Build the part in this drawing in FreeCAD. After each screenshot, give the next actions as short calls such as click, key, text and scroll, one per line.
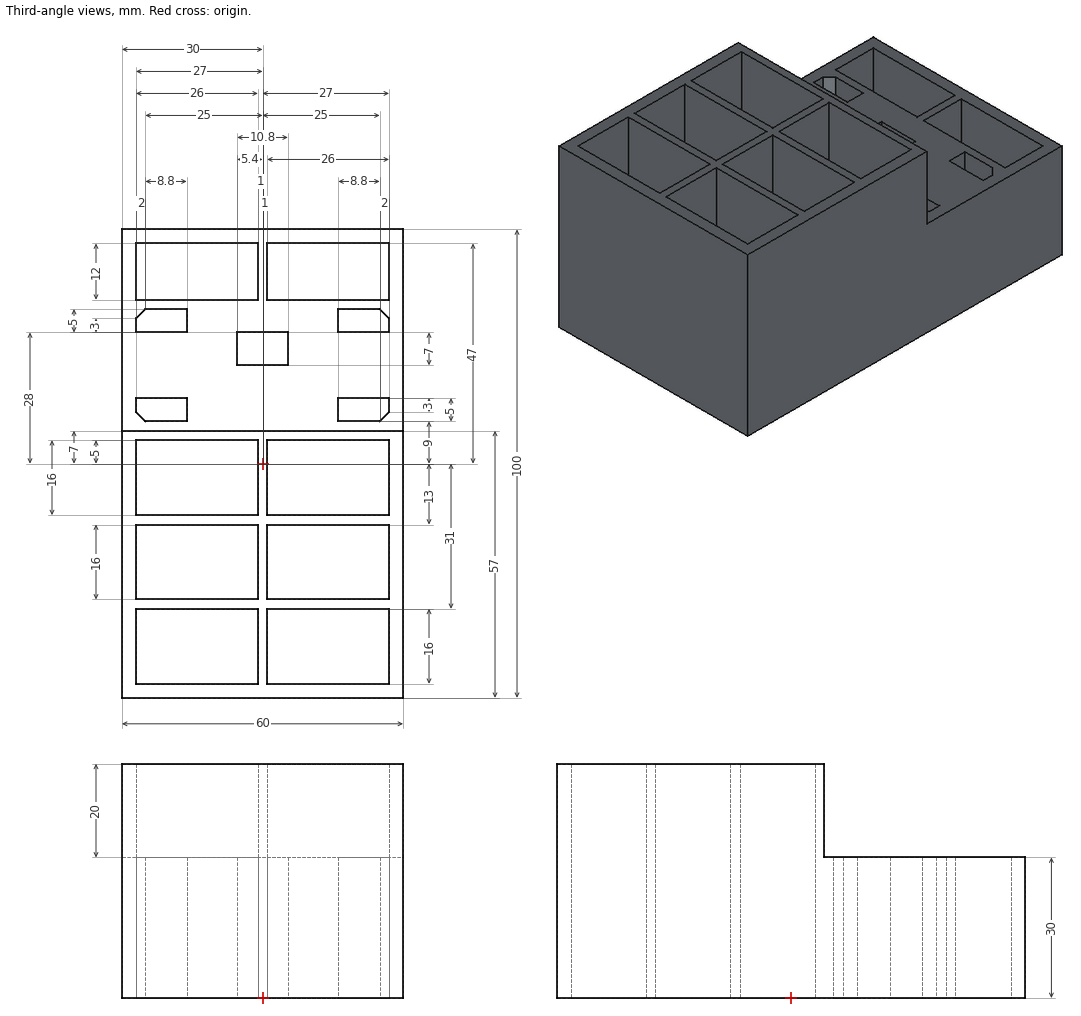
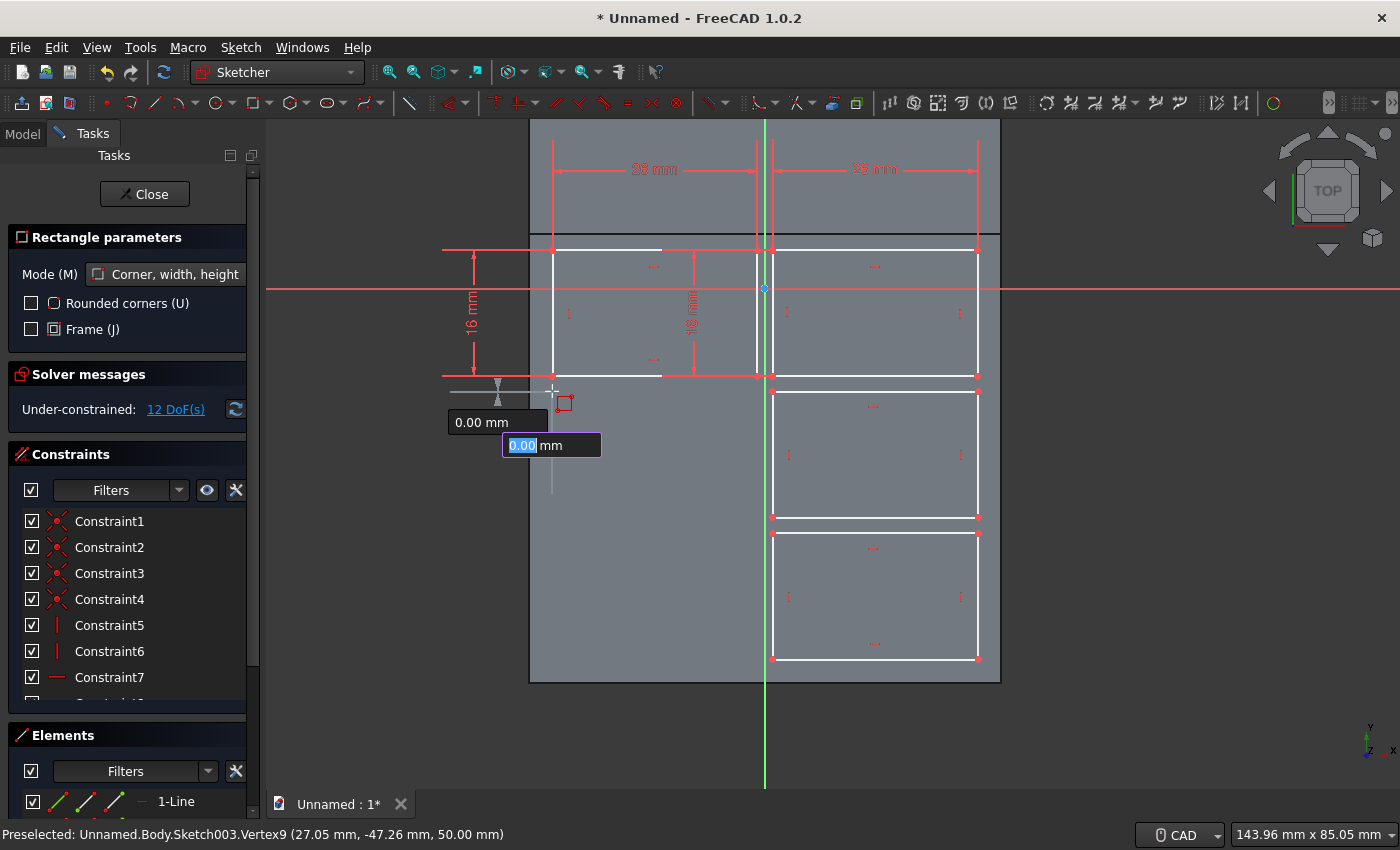
scroll(757, 517, up, 4)
move(756, 517)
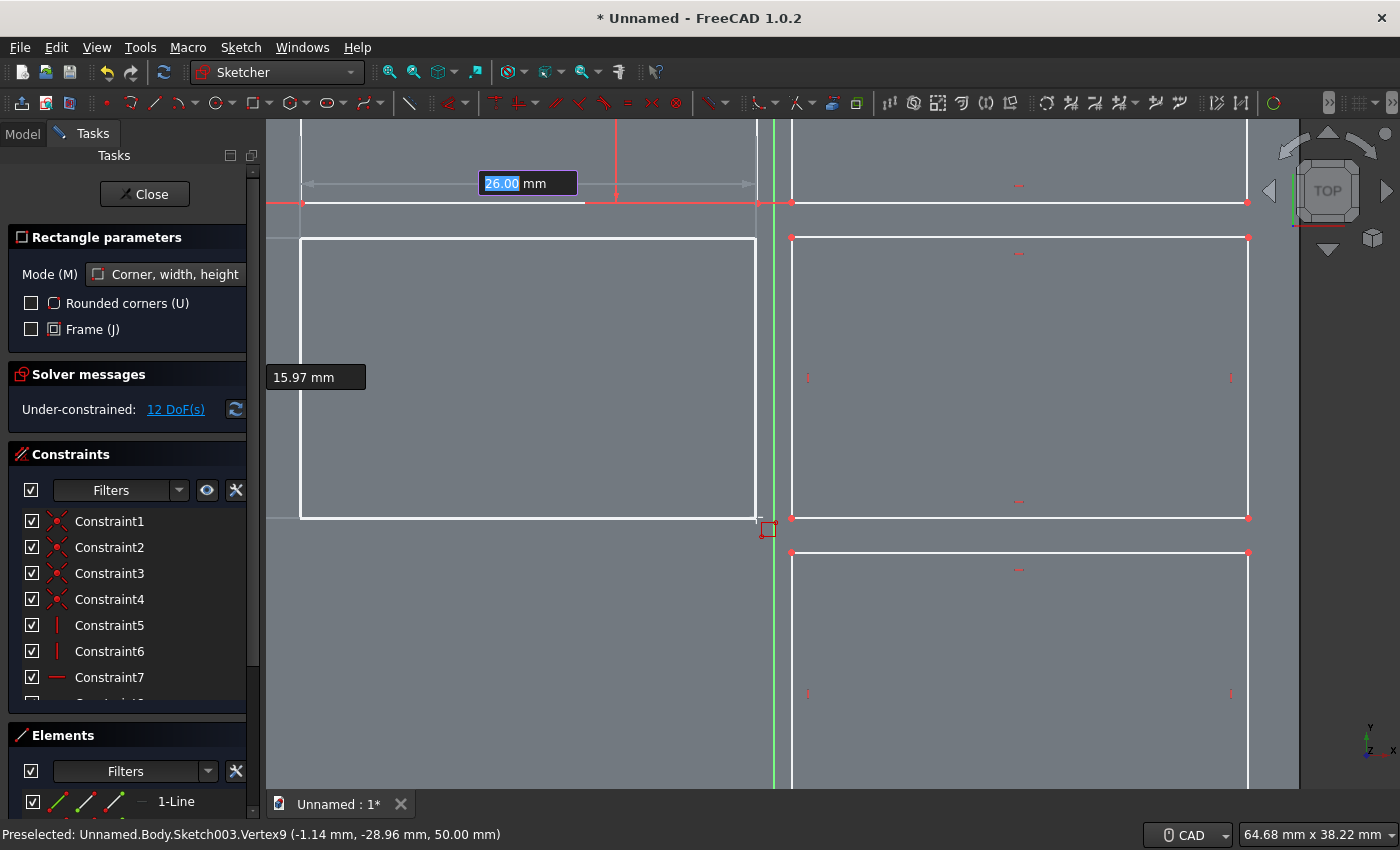
text(26)
key(Tab)
text(16)
key(Return)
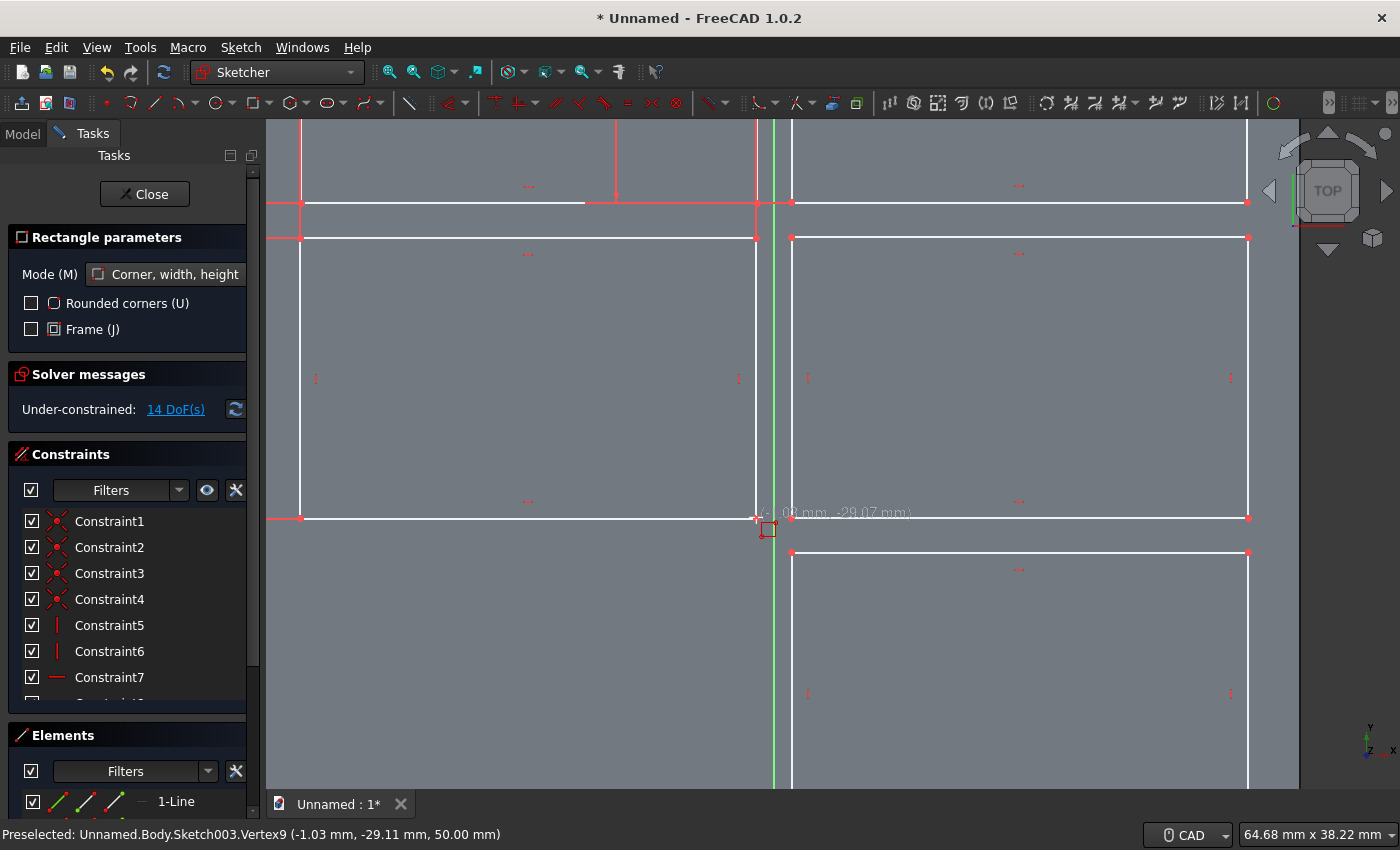
click(301, 552)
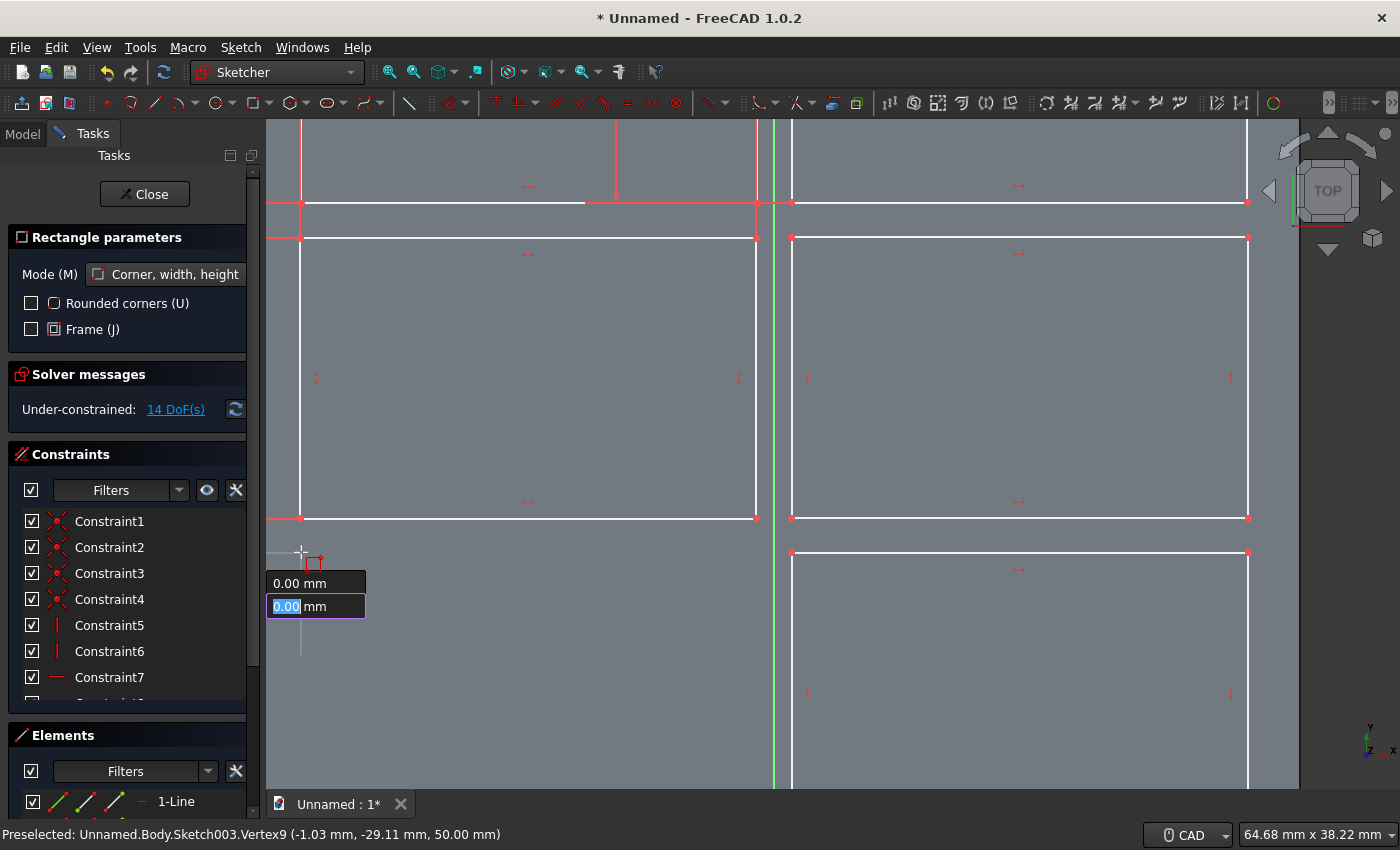
scroll(757, 517, down, 4)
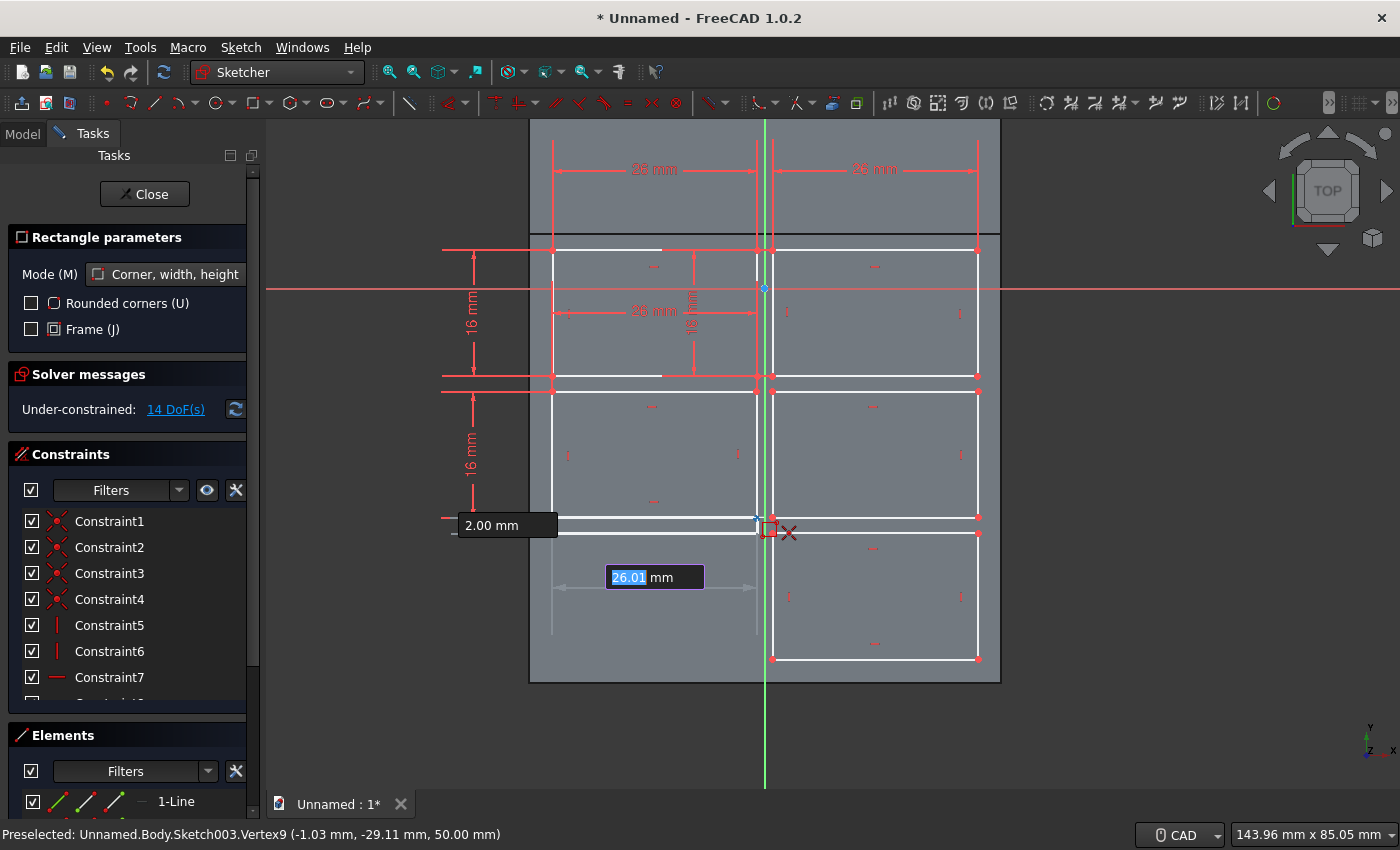
scroll(757, 659, up, 4)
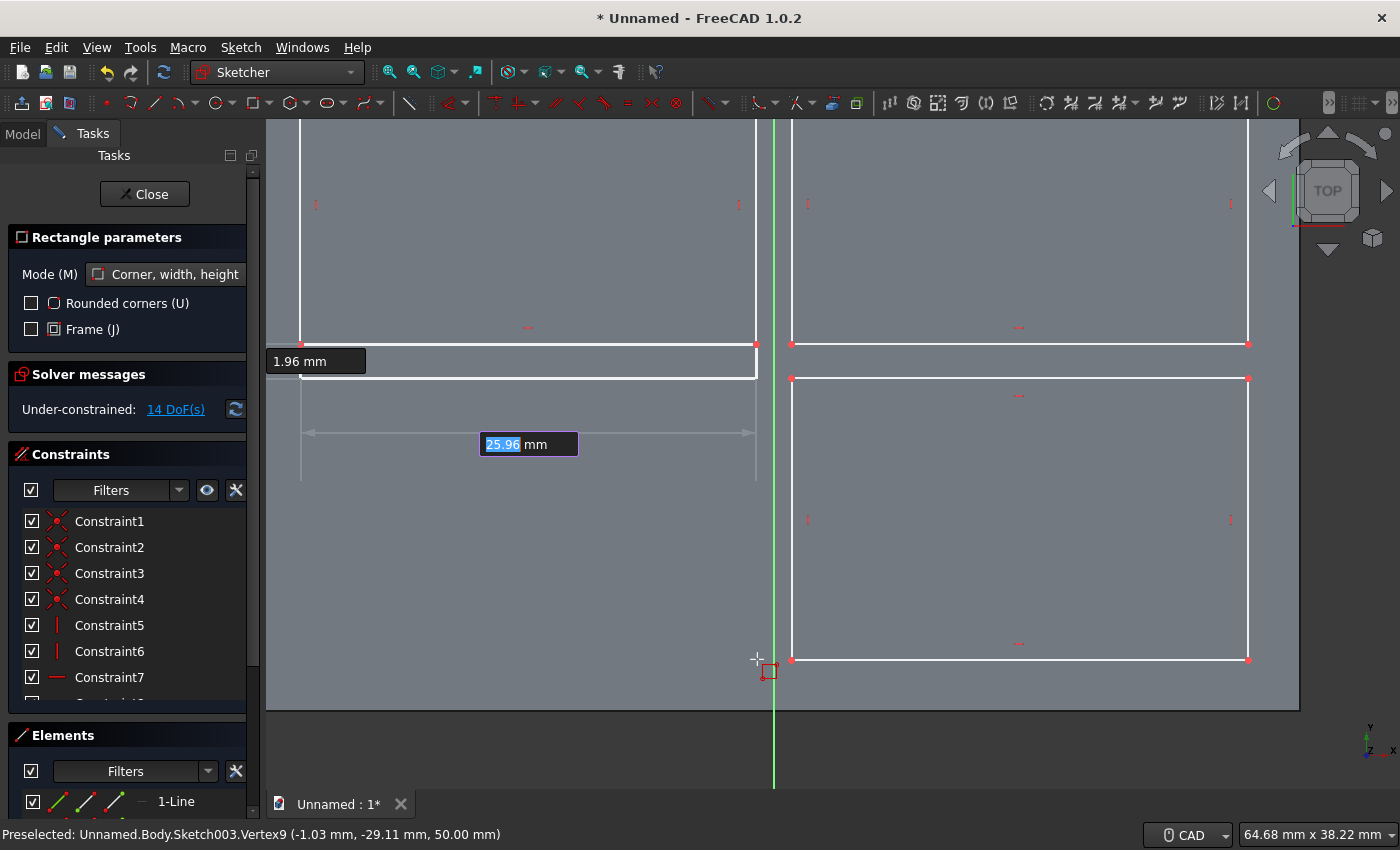
click(756, 658)
key(Escape)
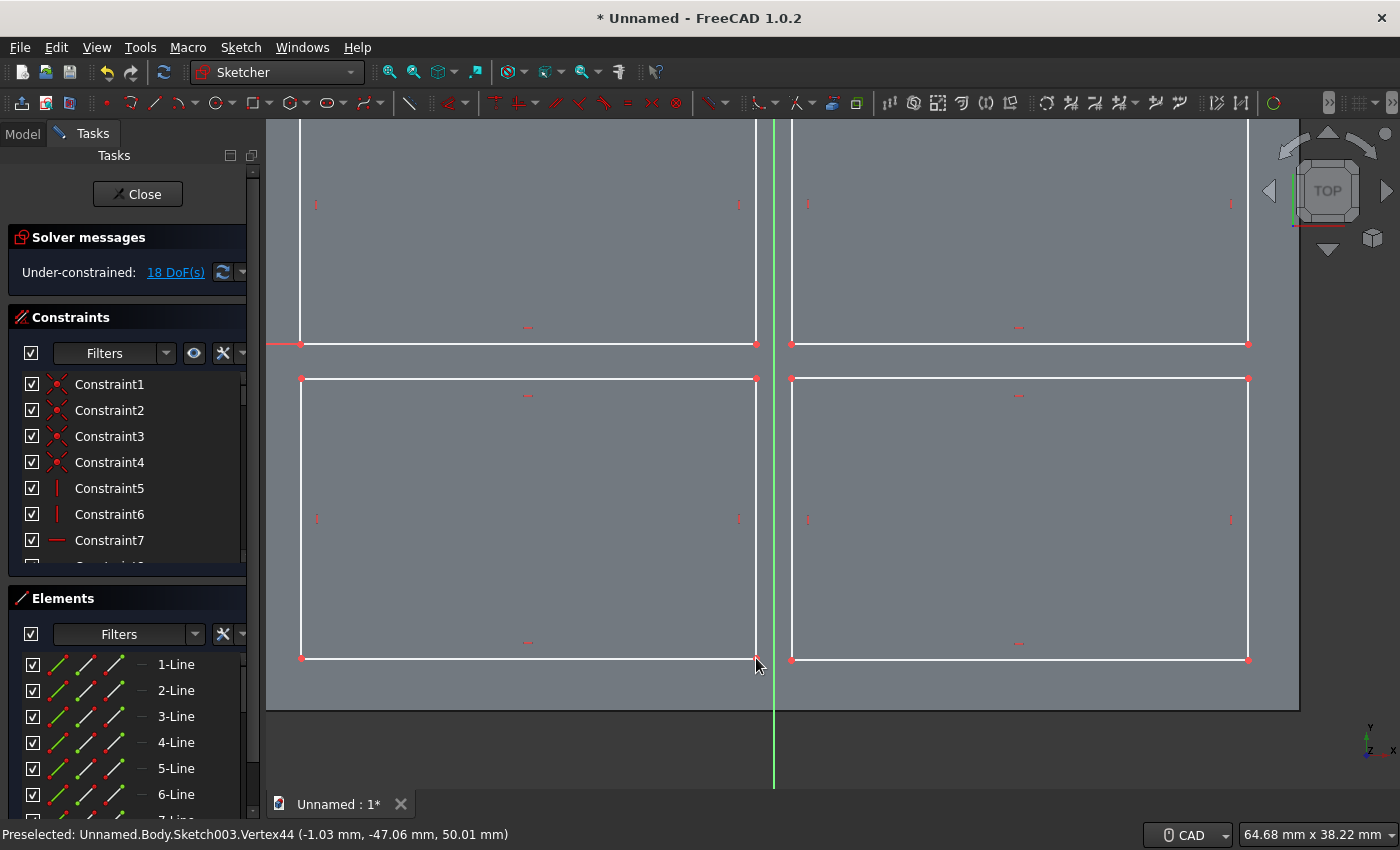
key(d)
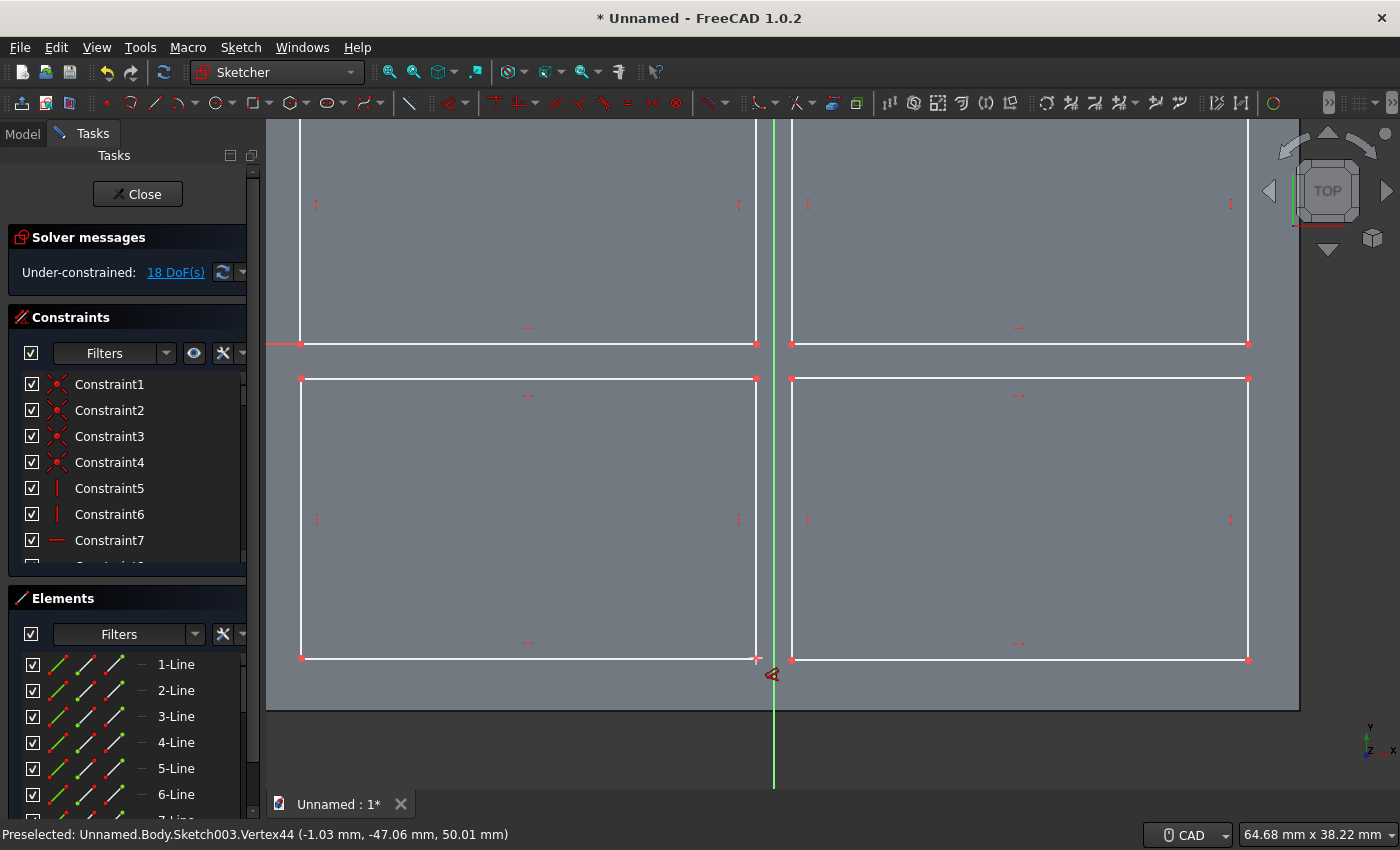
click(792, 147)
click(826, 246)